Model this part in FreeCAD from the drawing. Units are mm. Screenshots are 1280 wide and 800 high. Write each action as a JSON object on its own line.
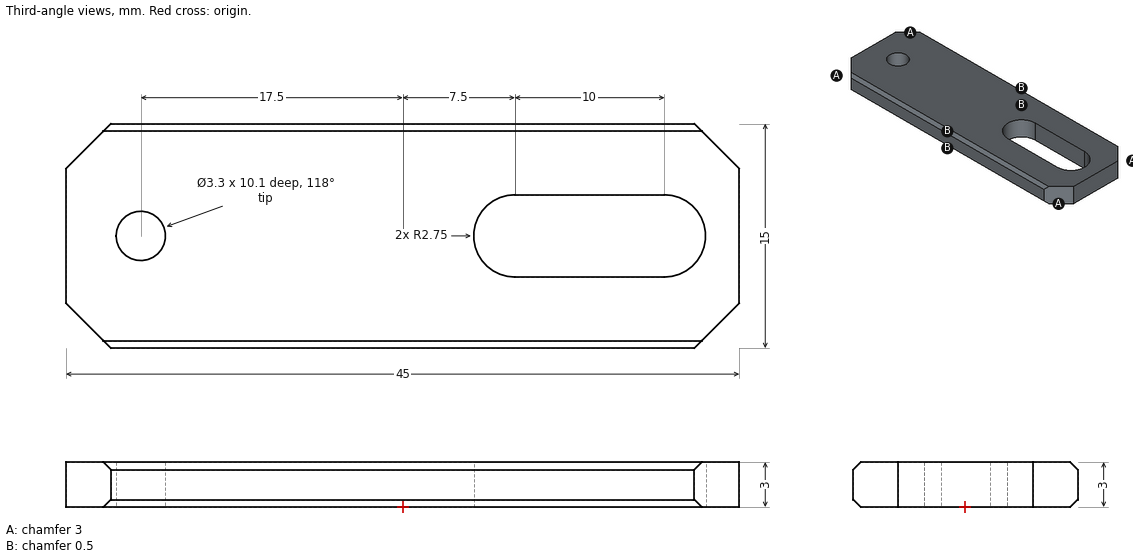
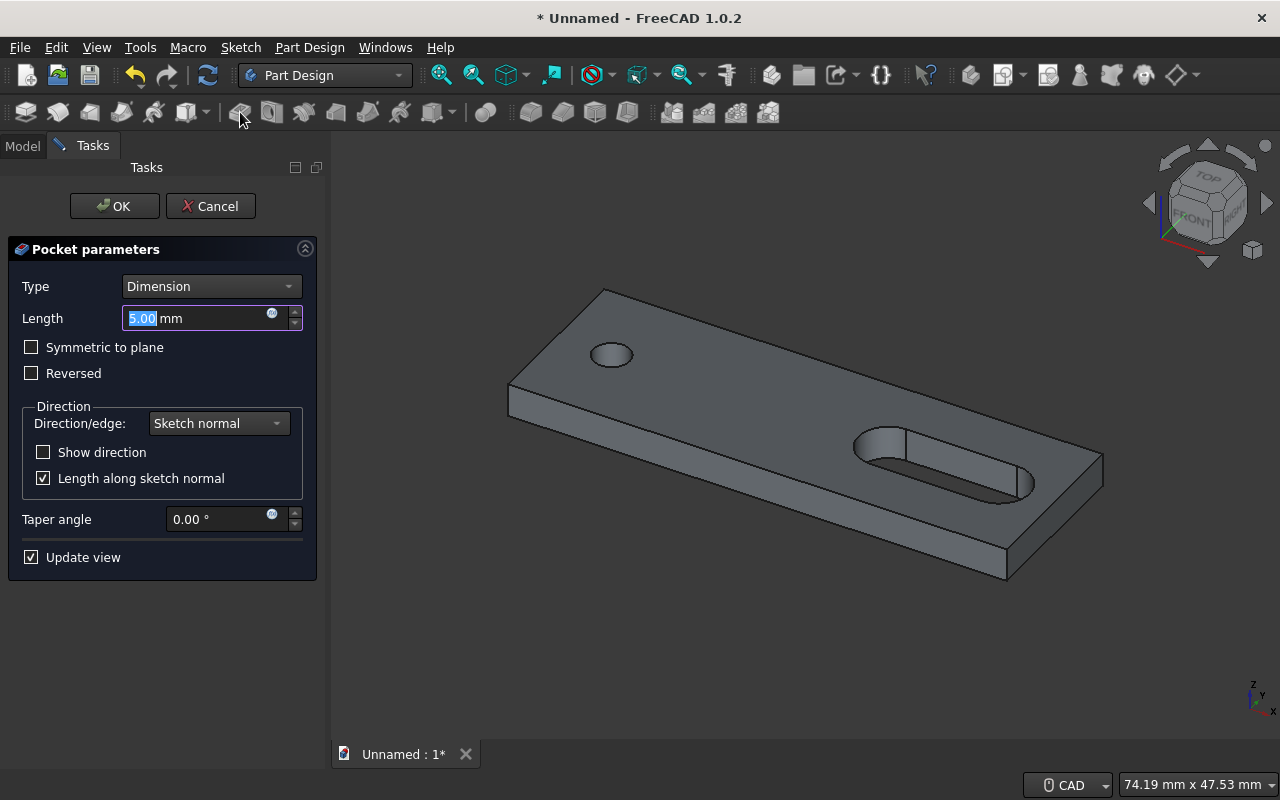
{"action": "type", "text": "3"}
{"action": "key", "text": "Tab"}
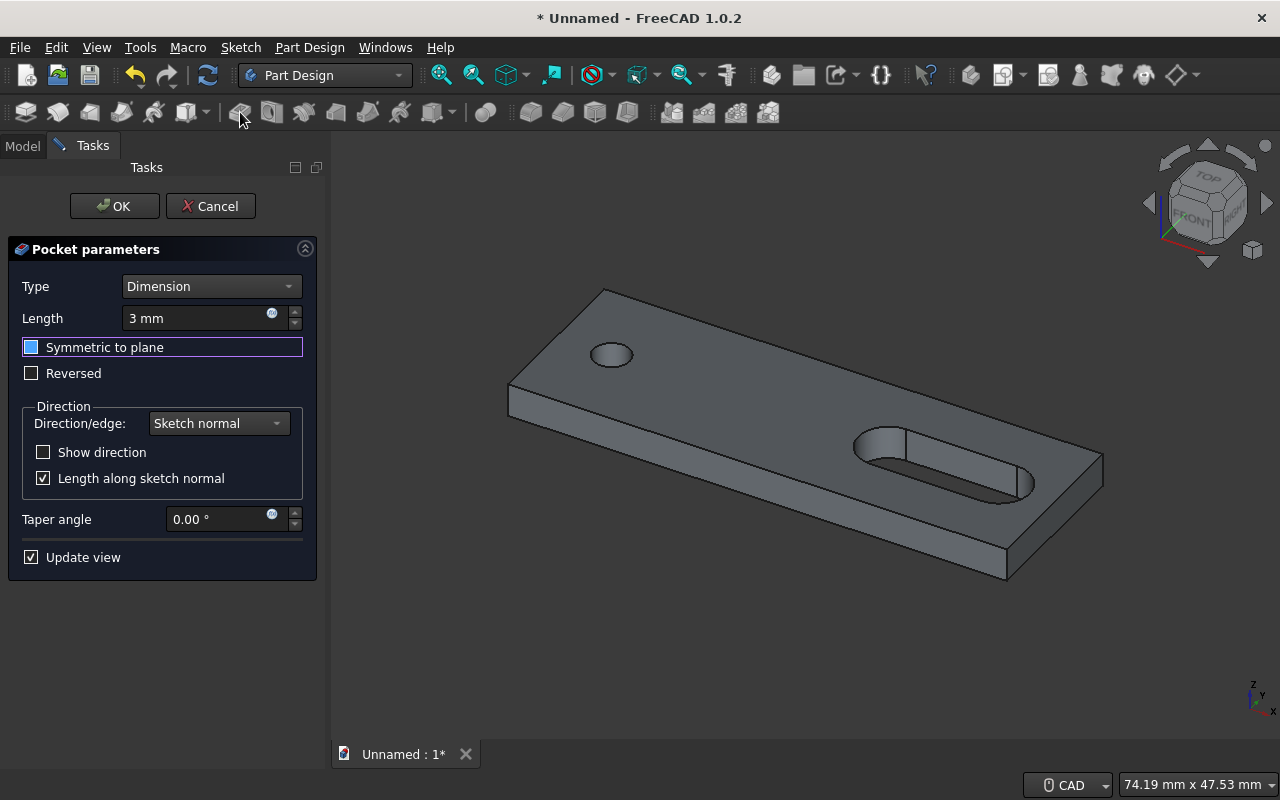
{"action": "left_click", "coordinate": [115, 206]}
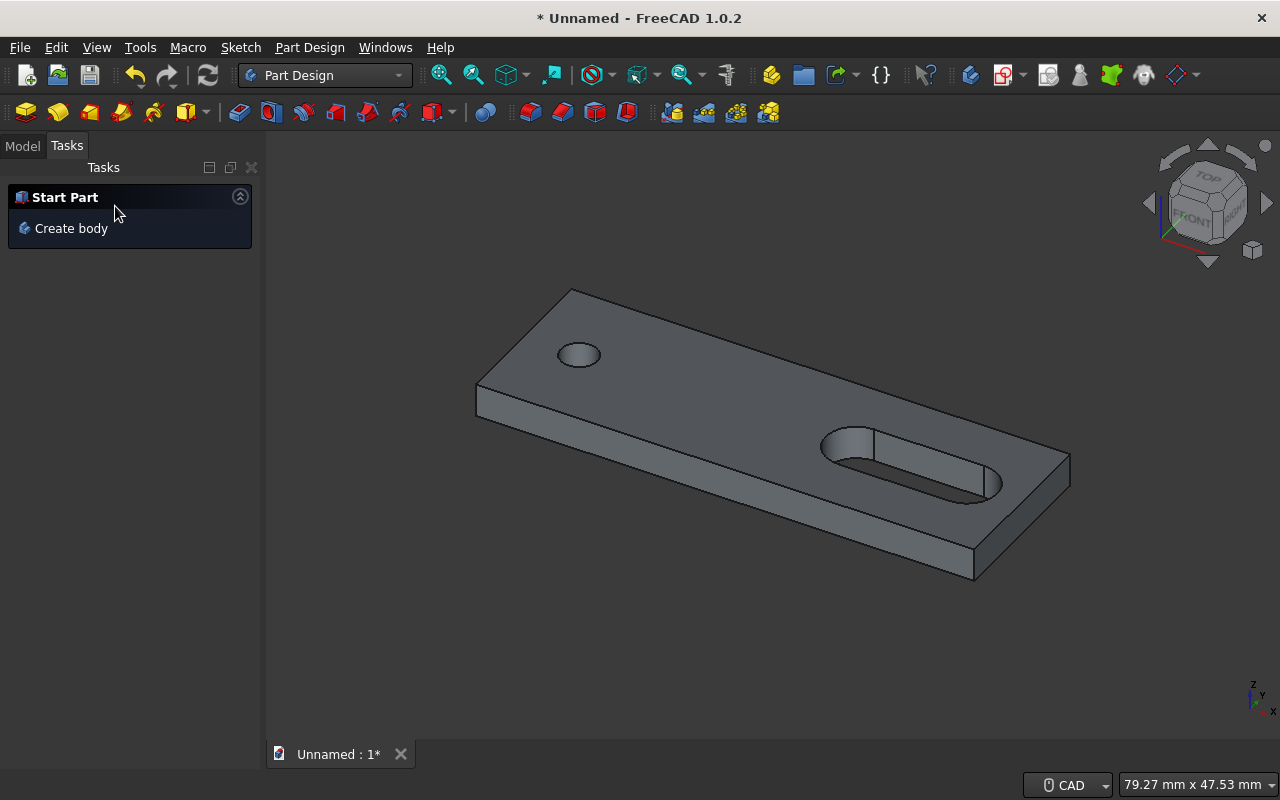
{"action": "left_click", "coordinate": [974, 564]}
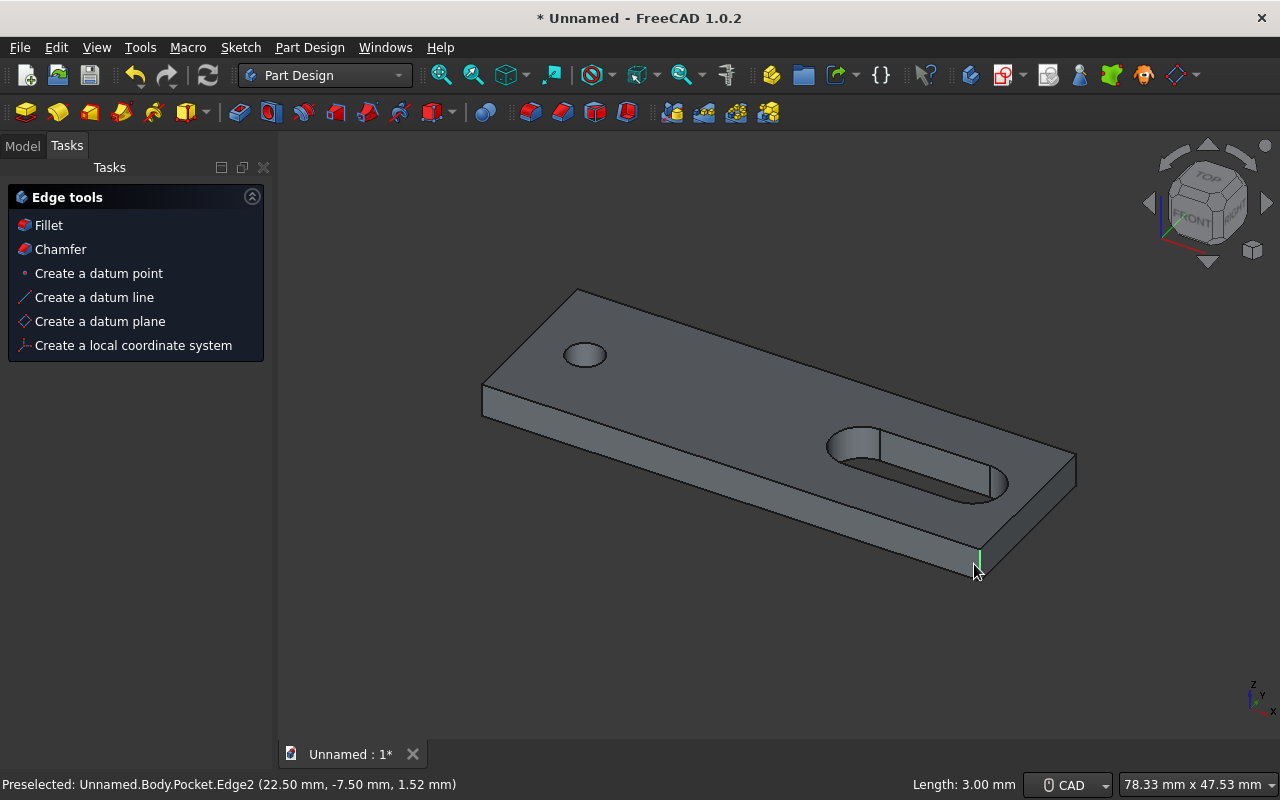
{"action": "key", "text": "0"}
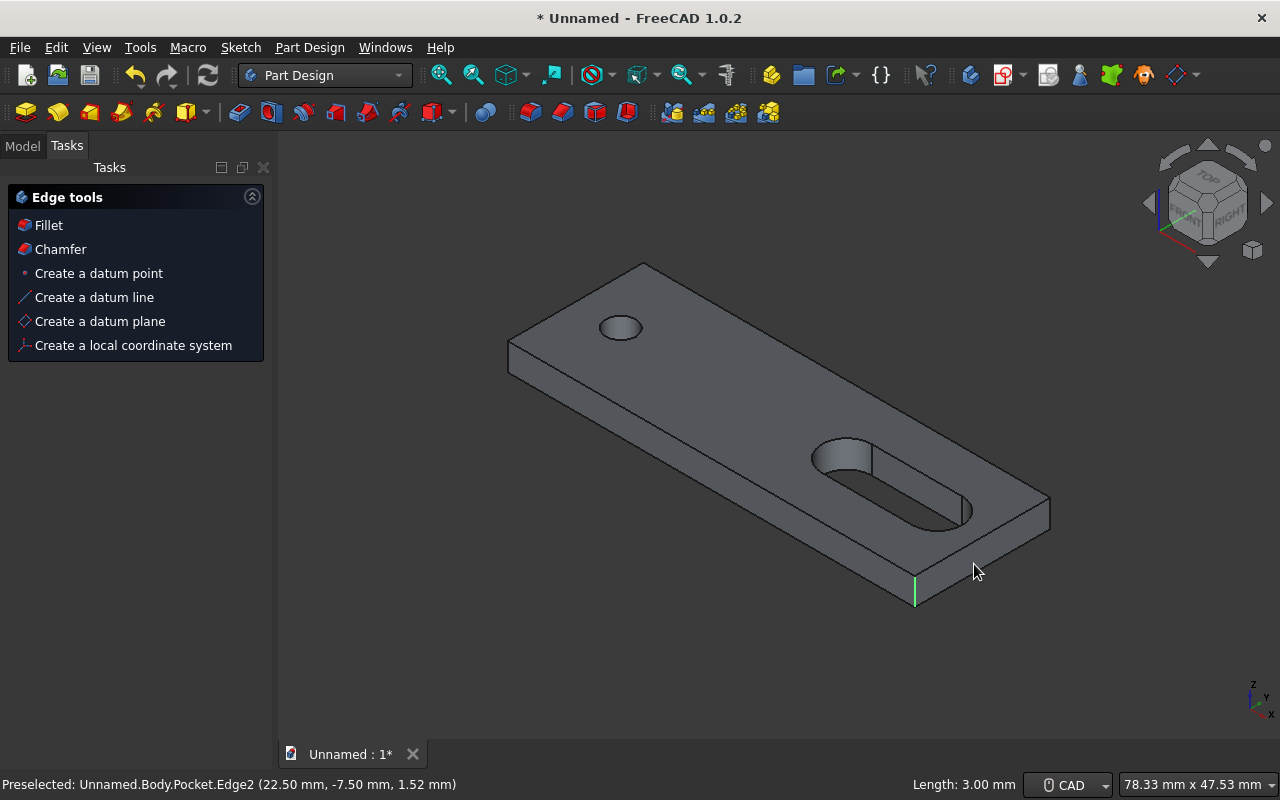
{"action": "key", "text": "2"}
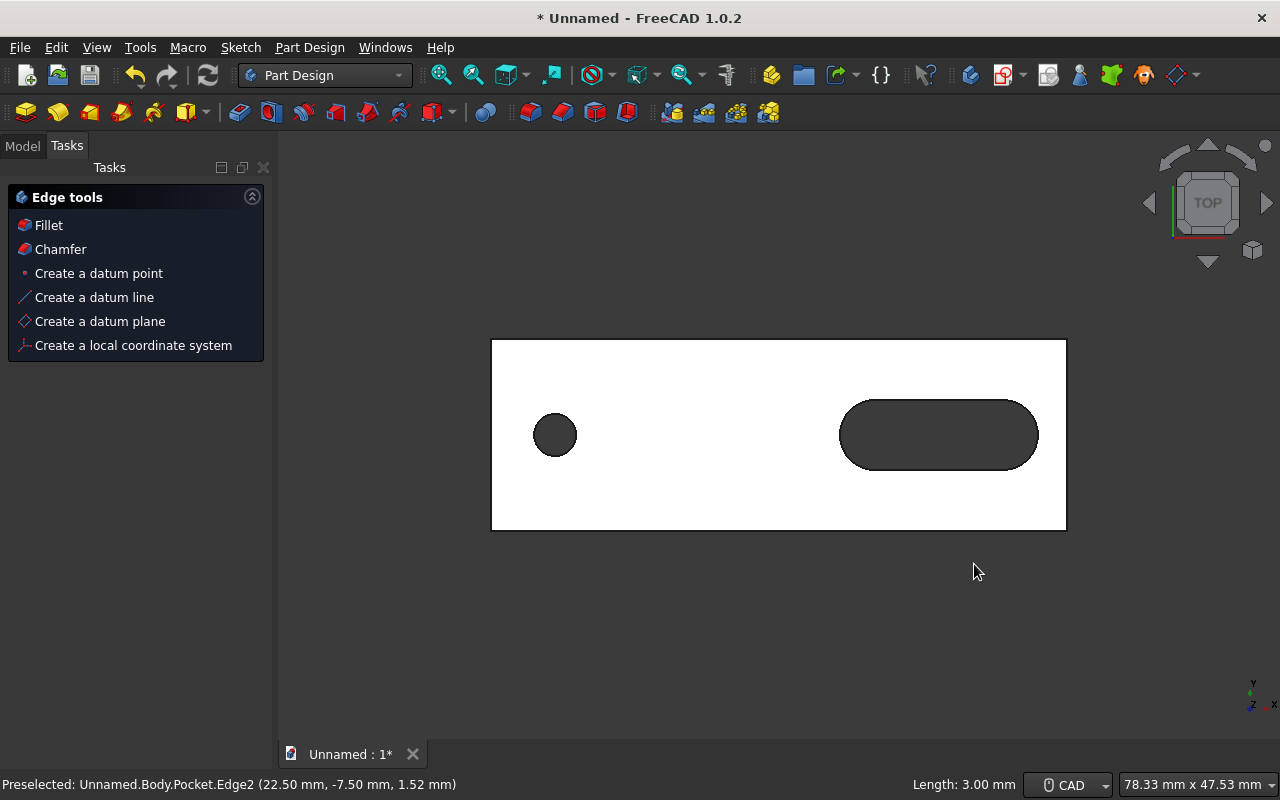
{"action": "key", "text": "1"}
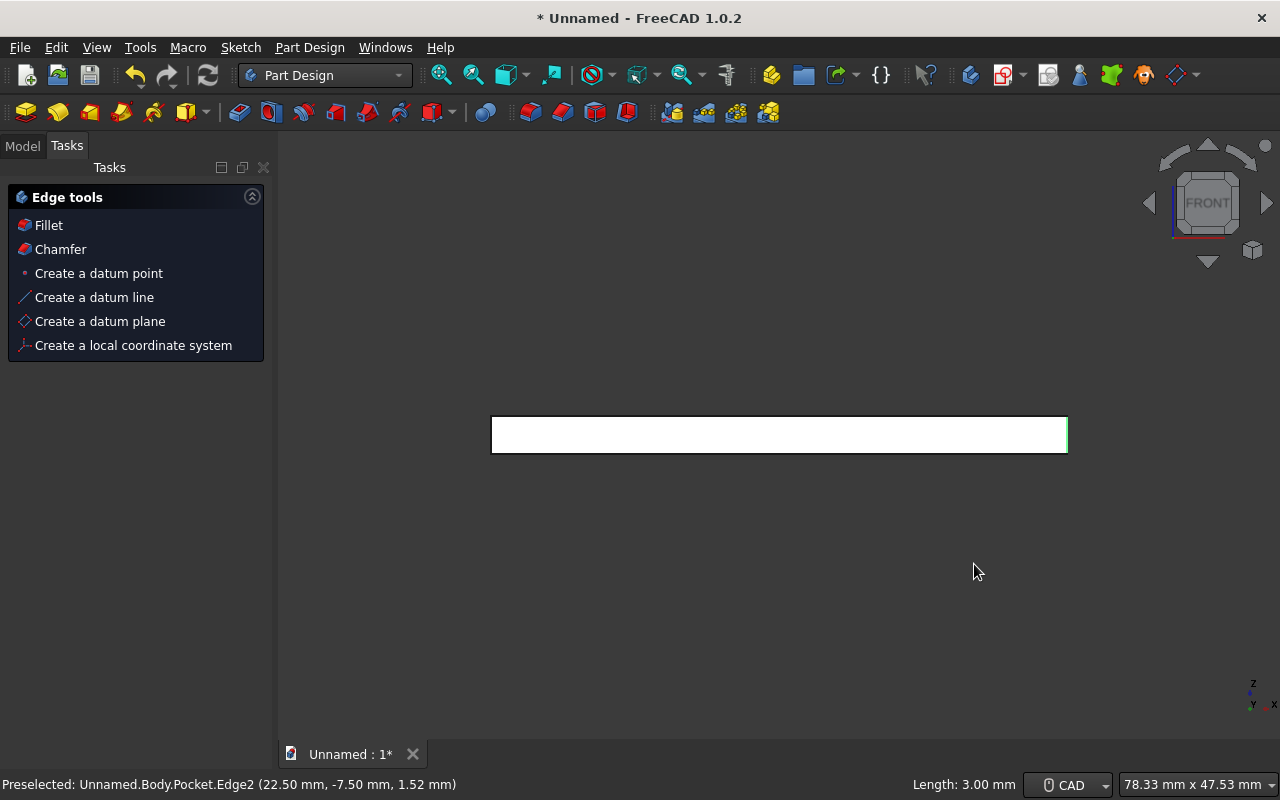
{"action": "left_click", "coordinate": [491, 434], "text": "ctrl"}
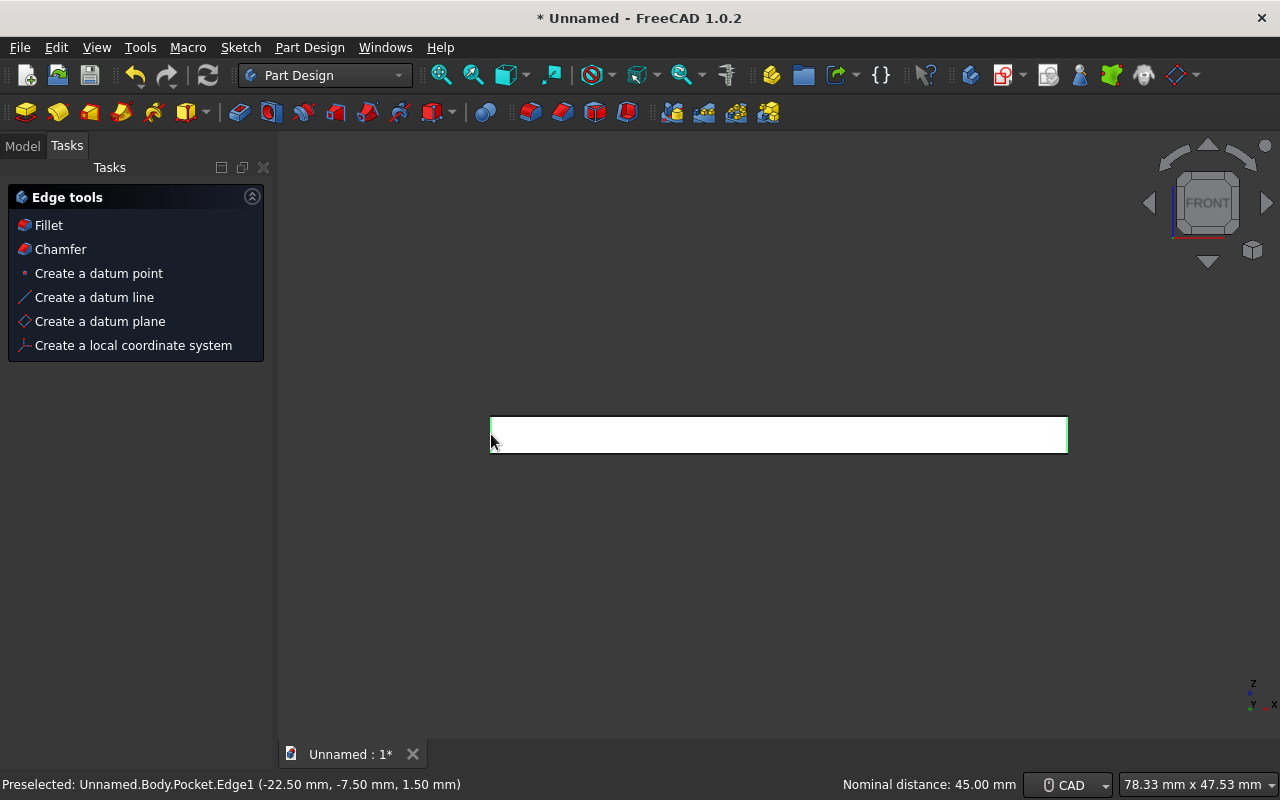
{"action": "key", "text": "3"}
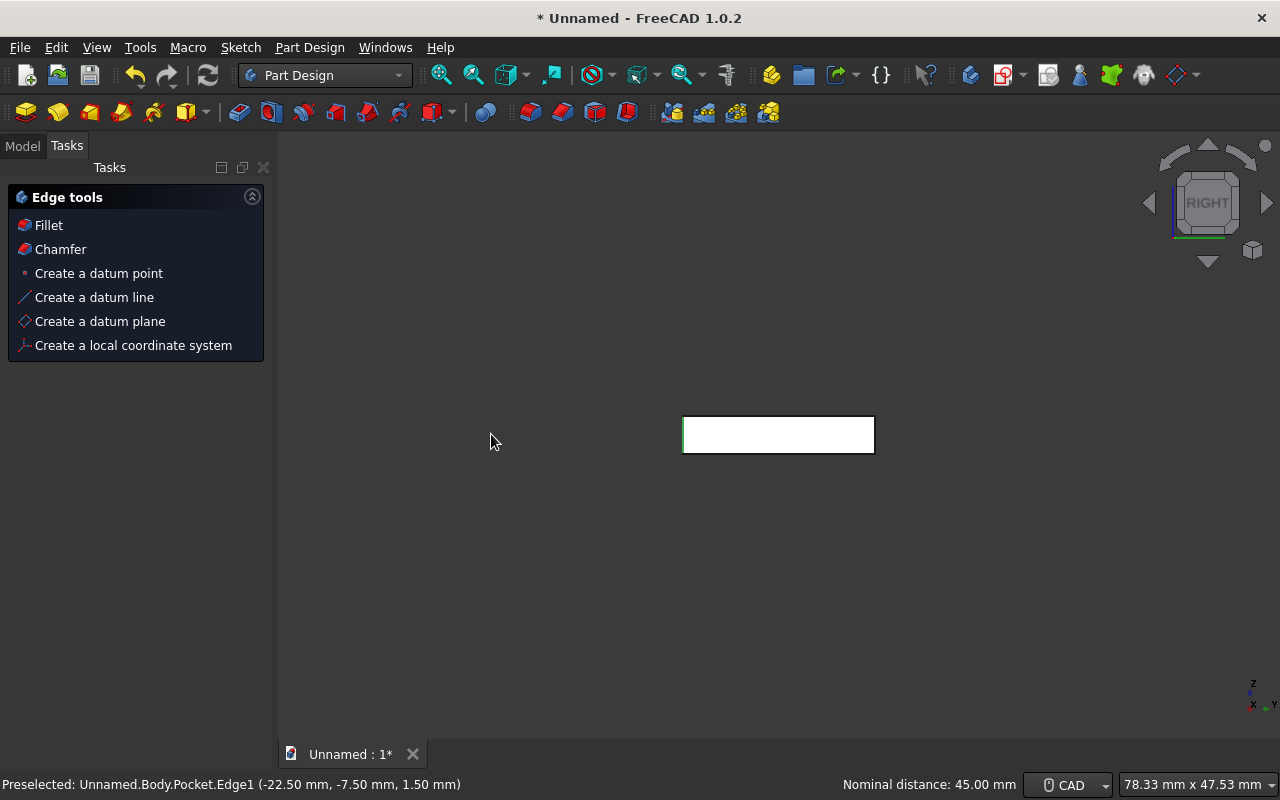
{"action": "left_click", "coordinate": [442, 76]}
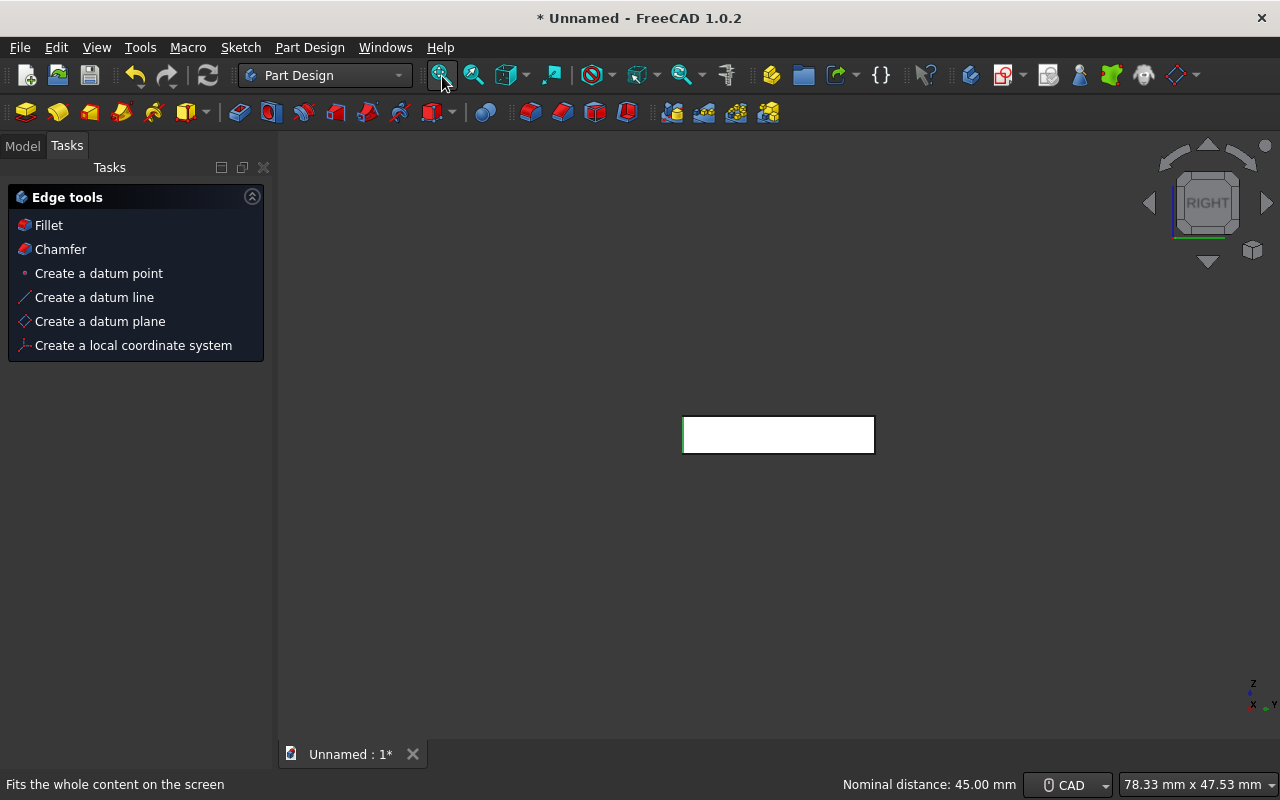
{"action": "left_click", "coordinate": [875, 434], "text": "ctrl"}